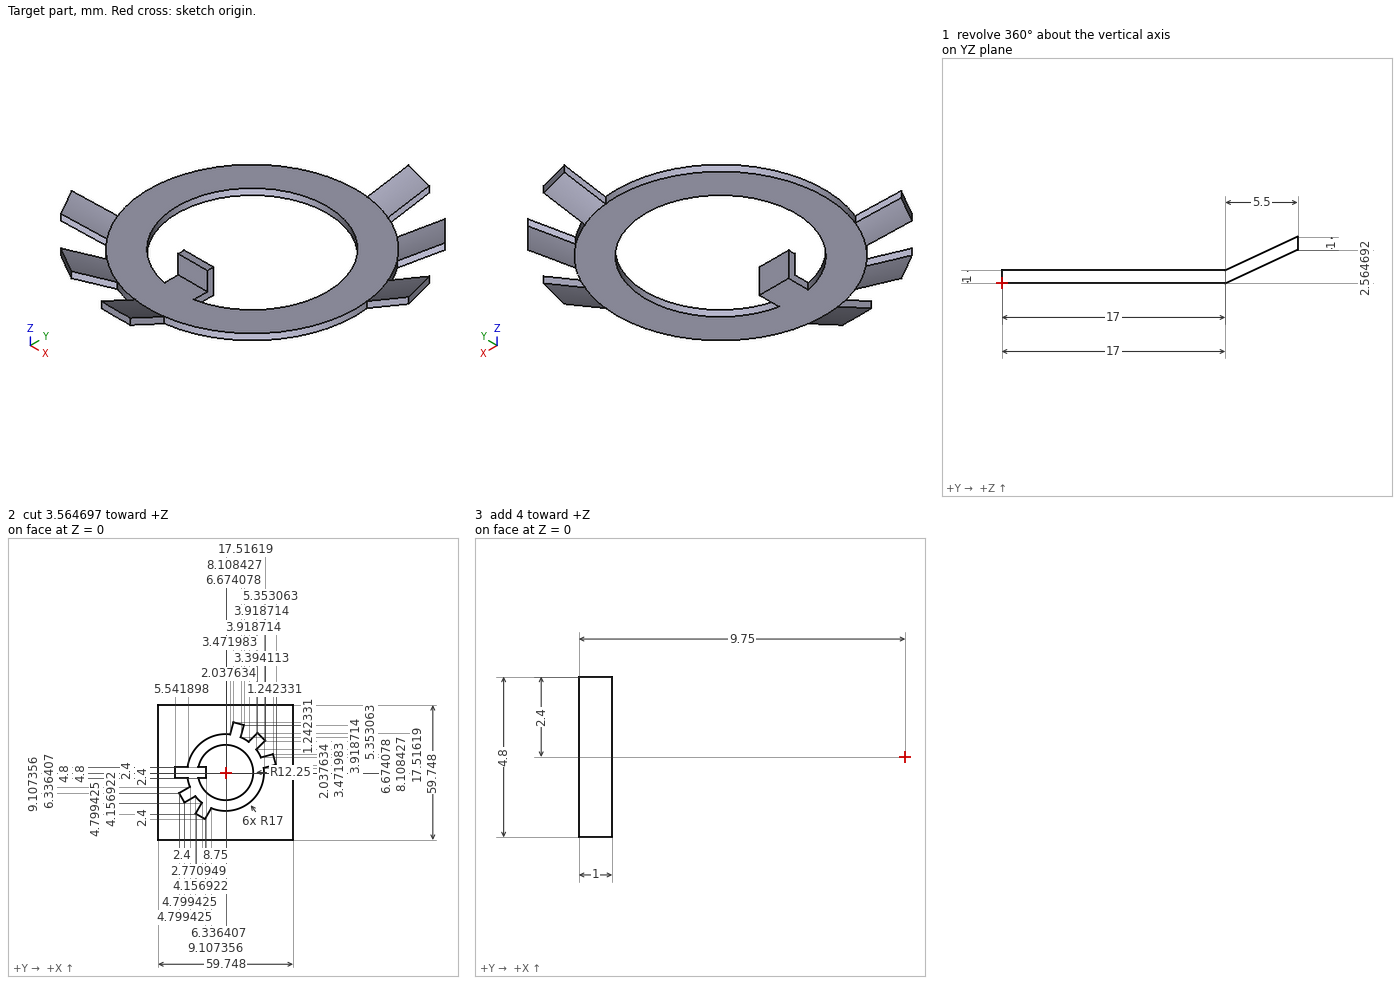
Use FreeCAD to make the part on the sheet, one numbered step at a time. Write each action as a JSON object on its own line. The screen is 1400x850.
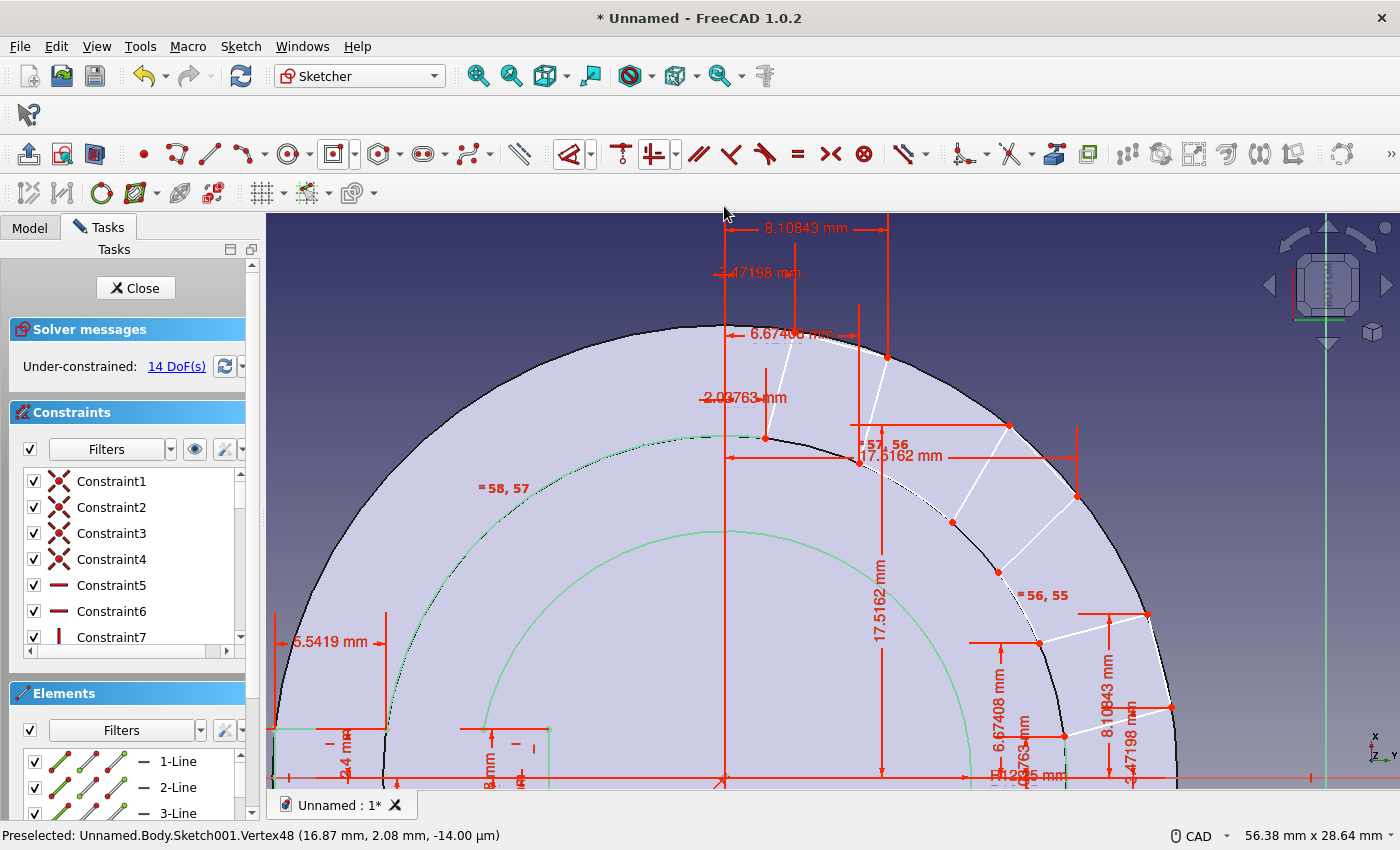
{"action": "scroll", "coordinate": [782, 382], "scroll_direction": "down", "scroll_amount": 6}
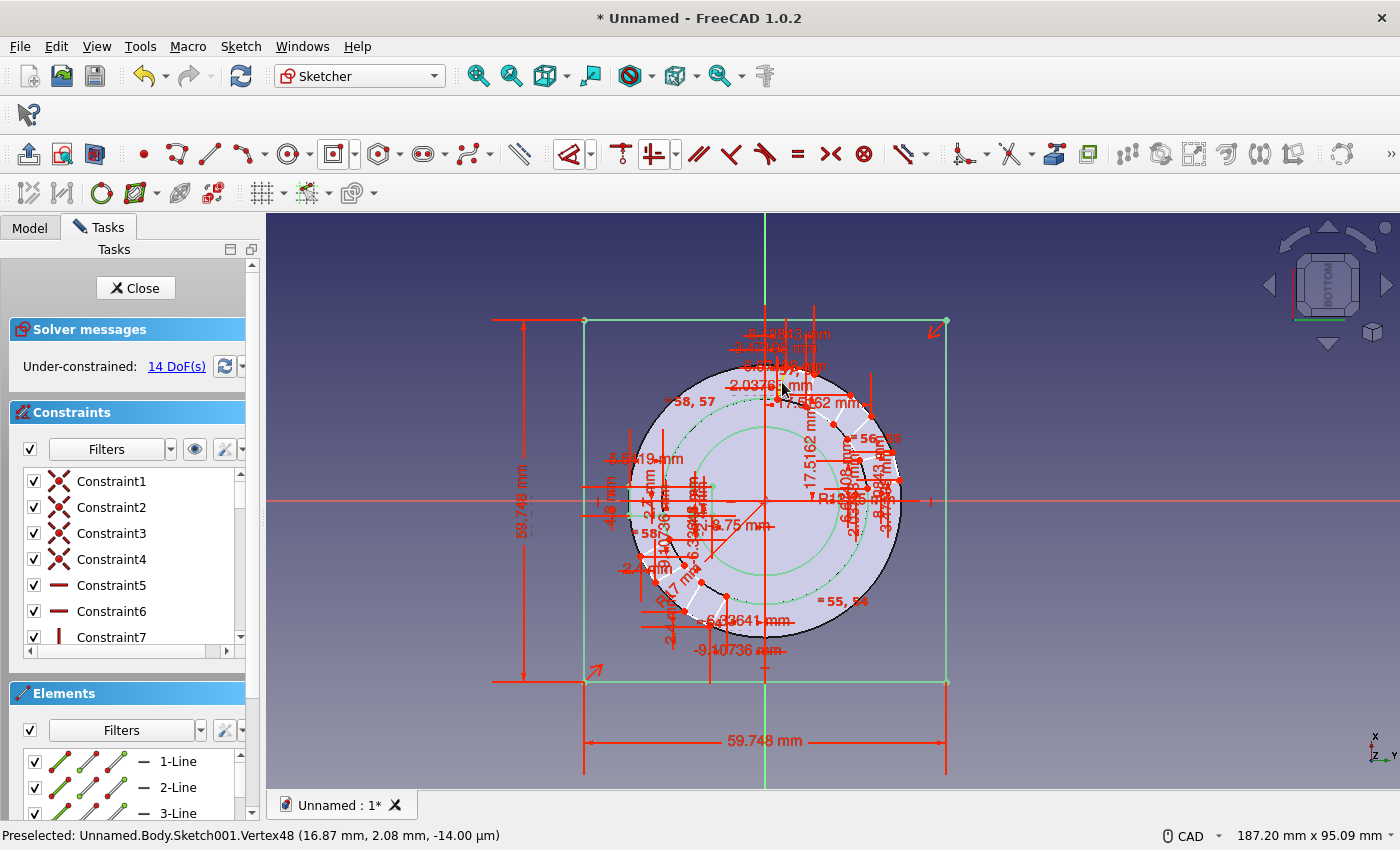
{"action": "scroll", "coordinate": [661, 545], "scroll_direction": "up", "scroll_amount": 2}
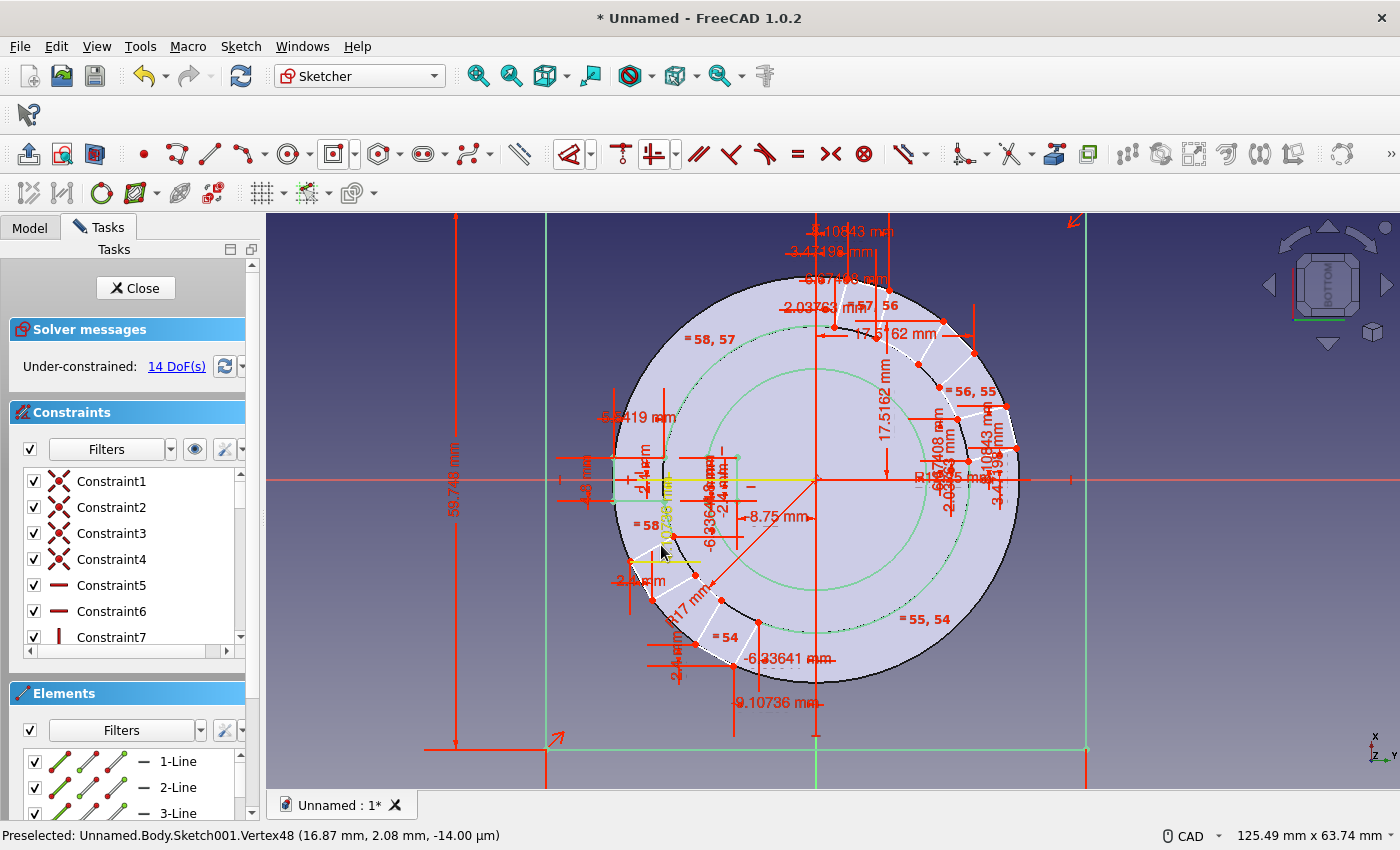
{"action": "left_click", "coordinate": [643, 554]}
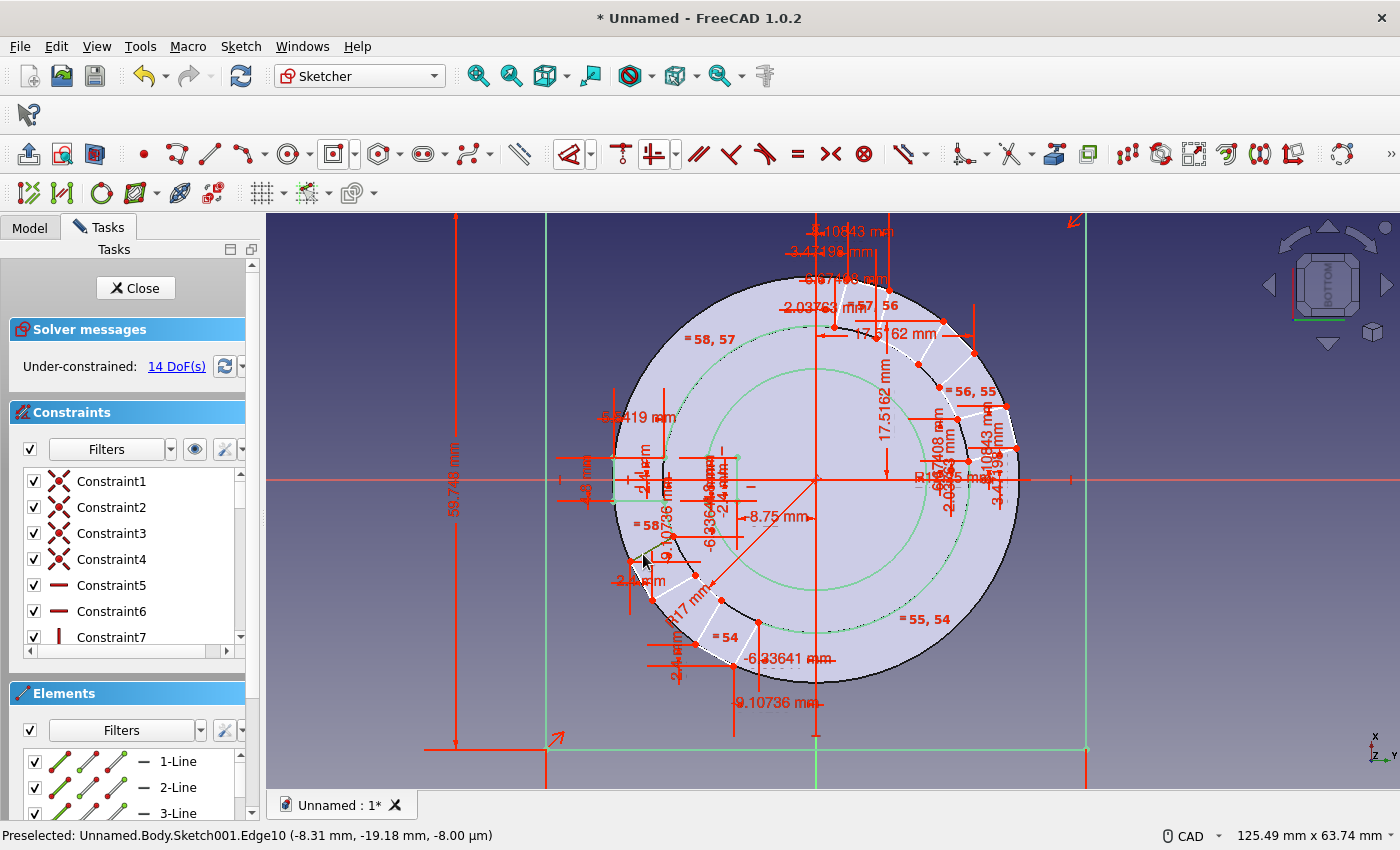
{"action": "left_click", "coordinate": [590, 154]}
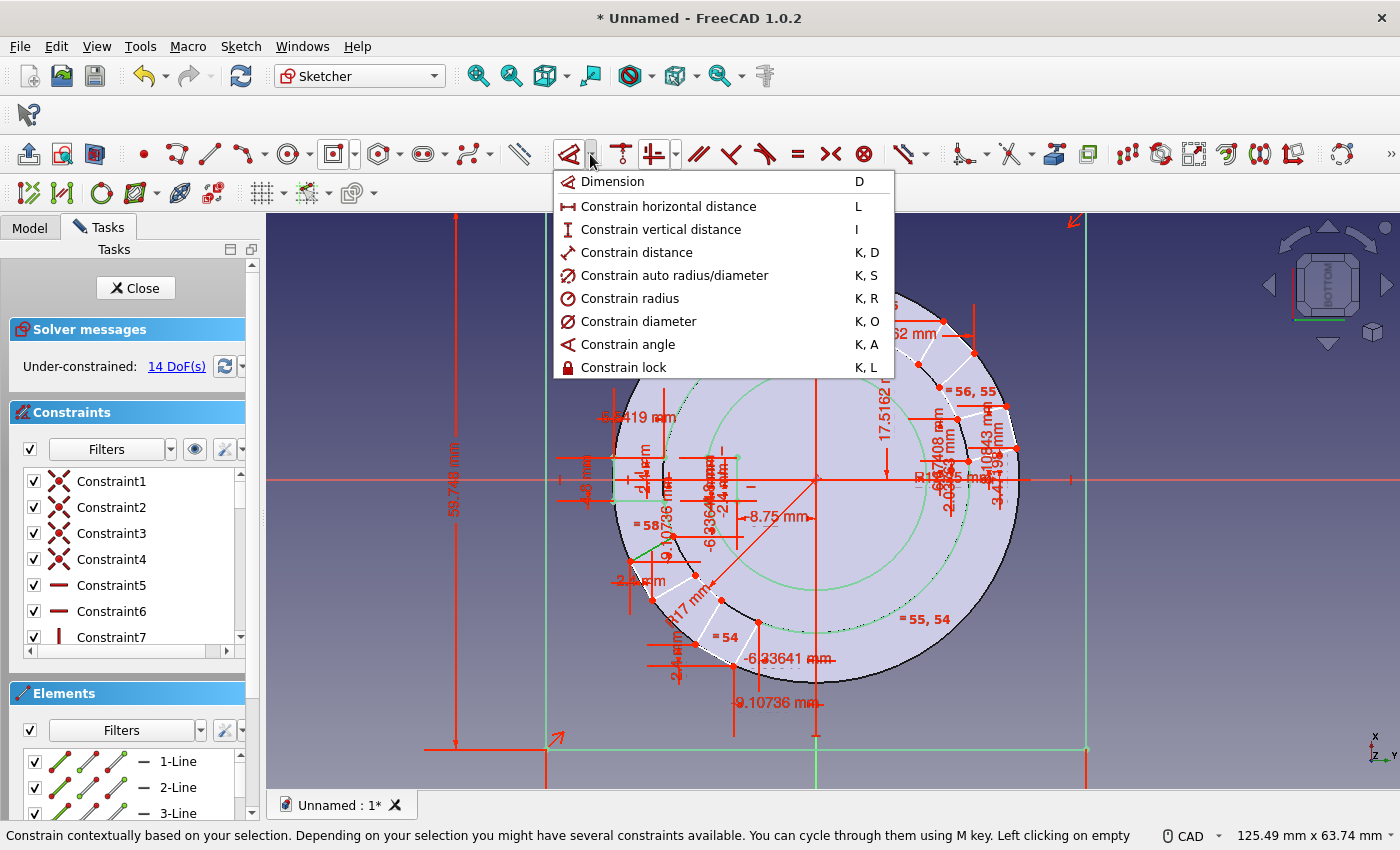
{"action": "left_click", "coordinate": [724, 206]}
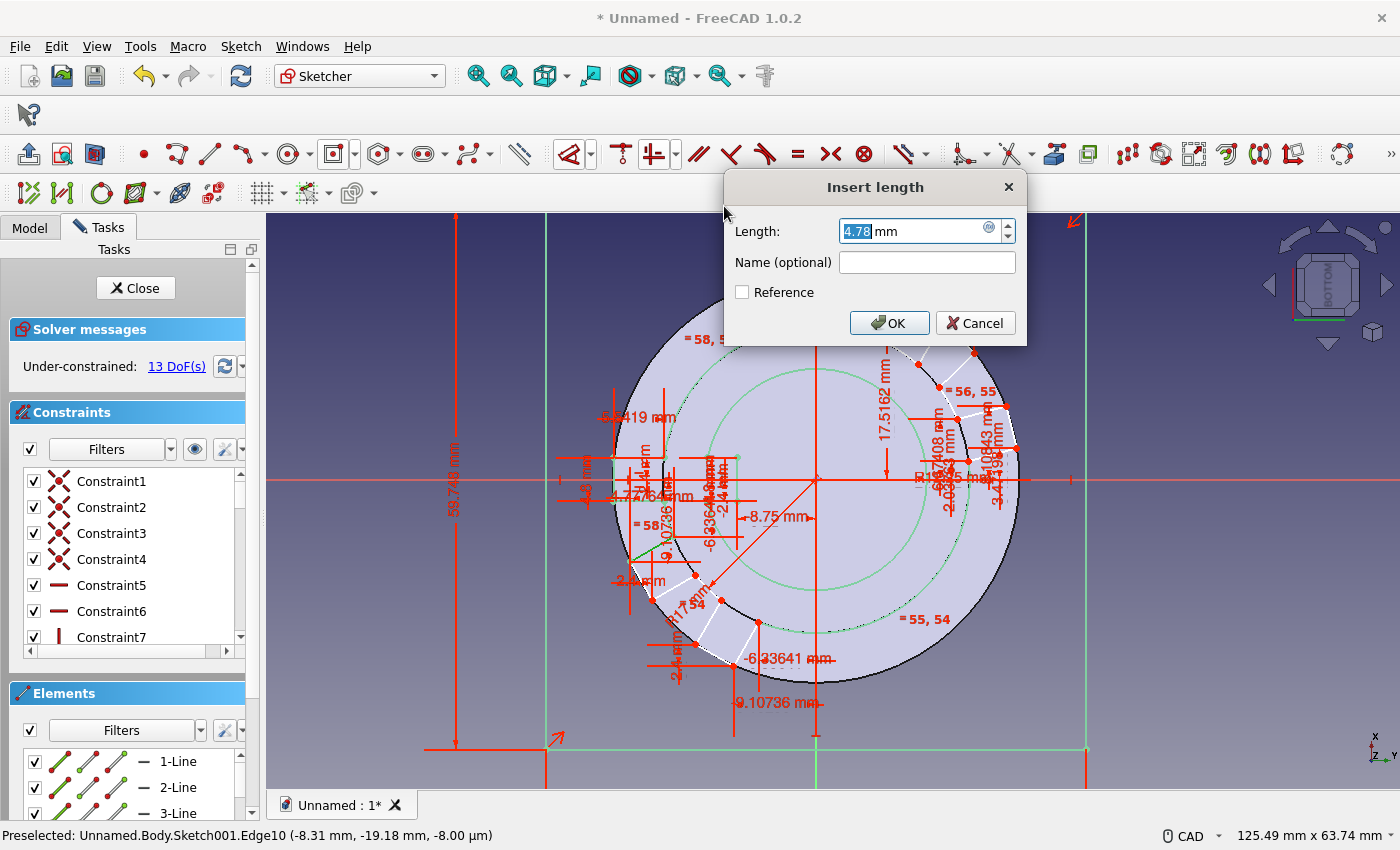
{"action": "type", "text": "4.799425"}
{"action": "key", "text": "Return"}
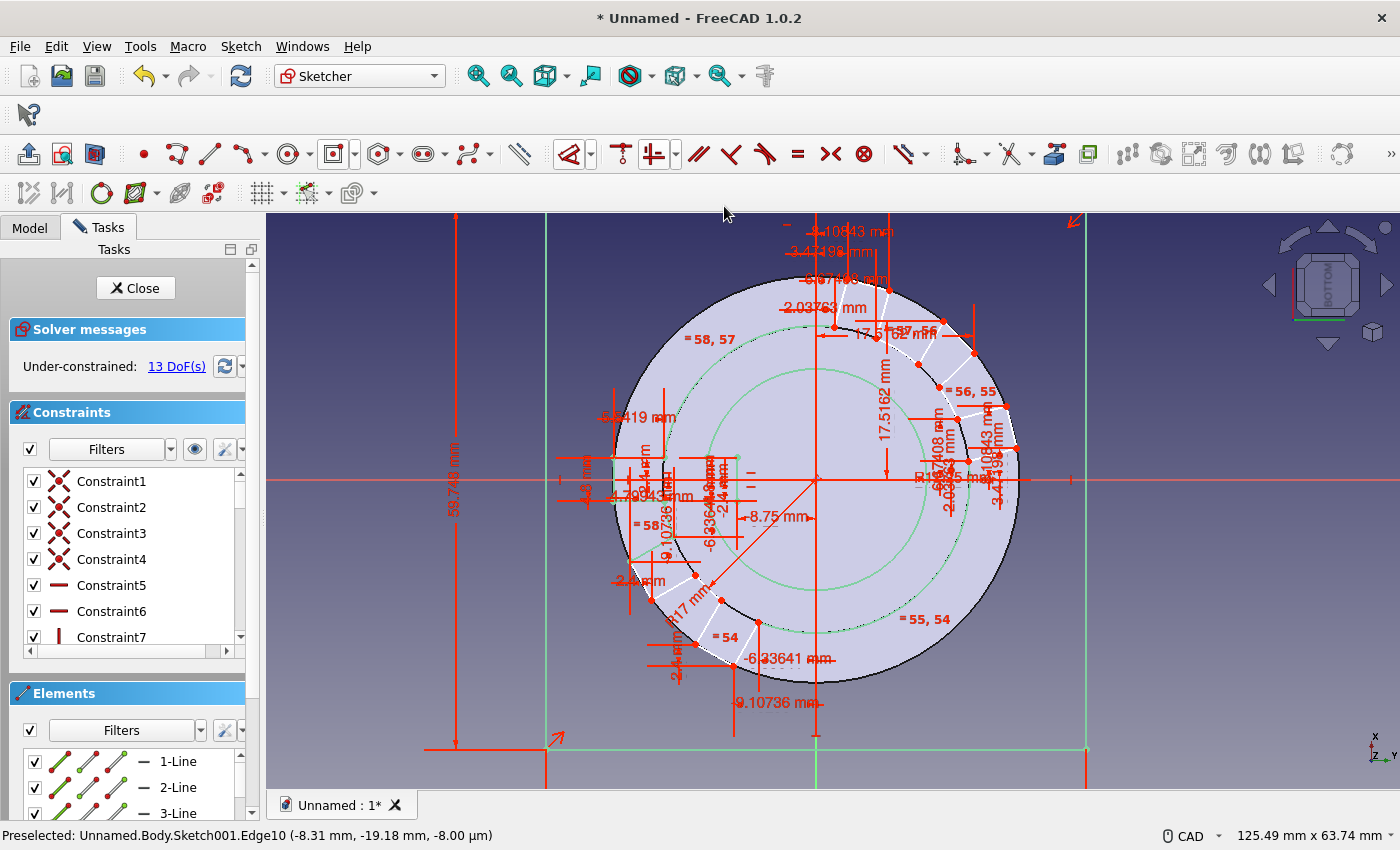
{"action": "left_click", "coordinate": [637, 573]}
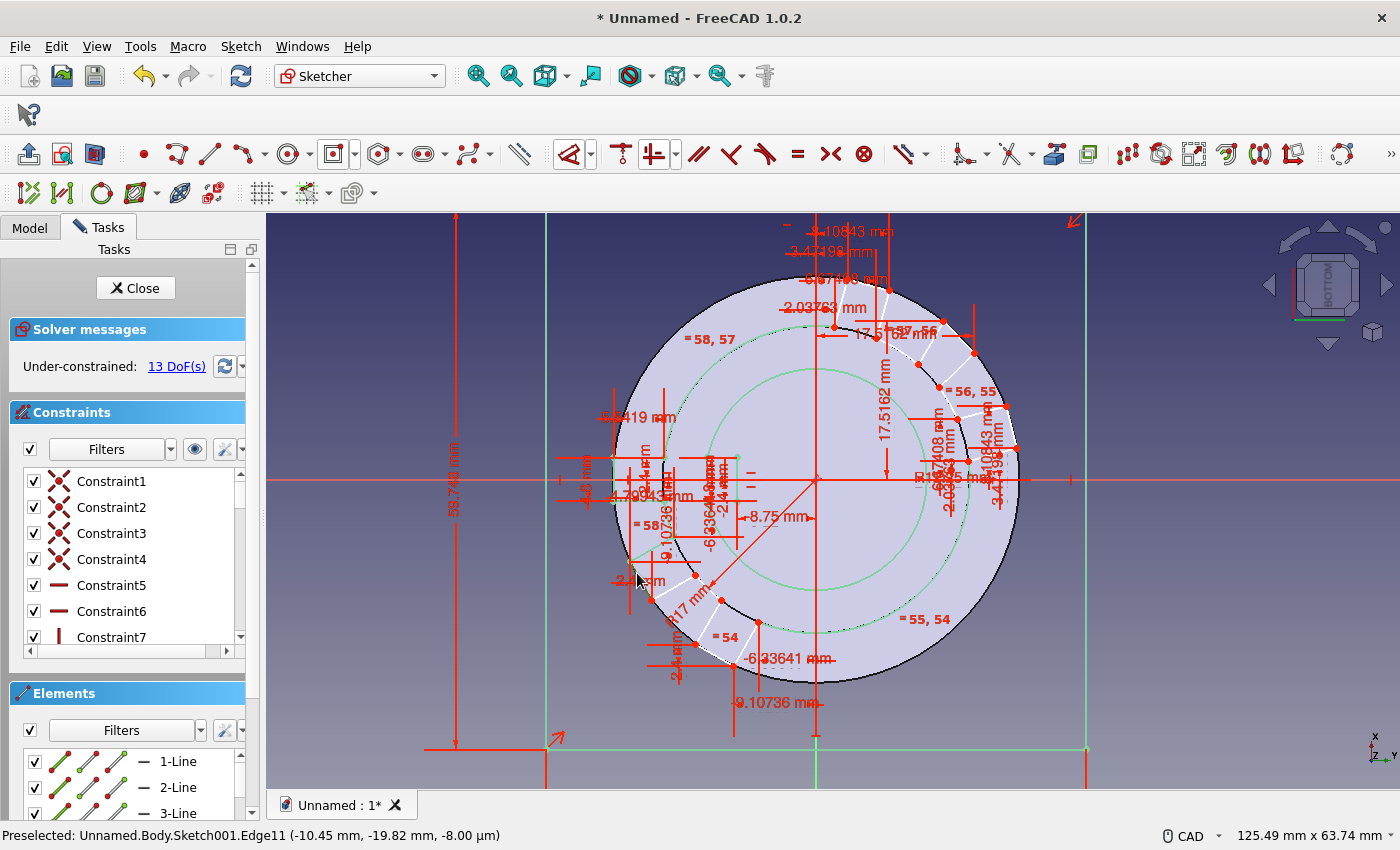
{"action": "key", "text": "i"}